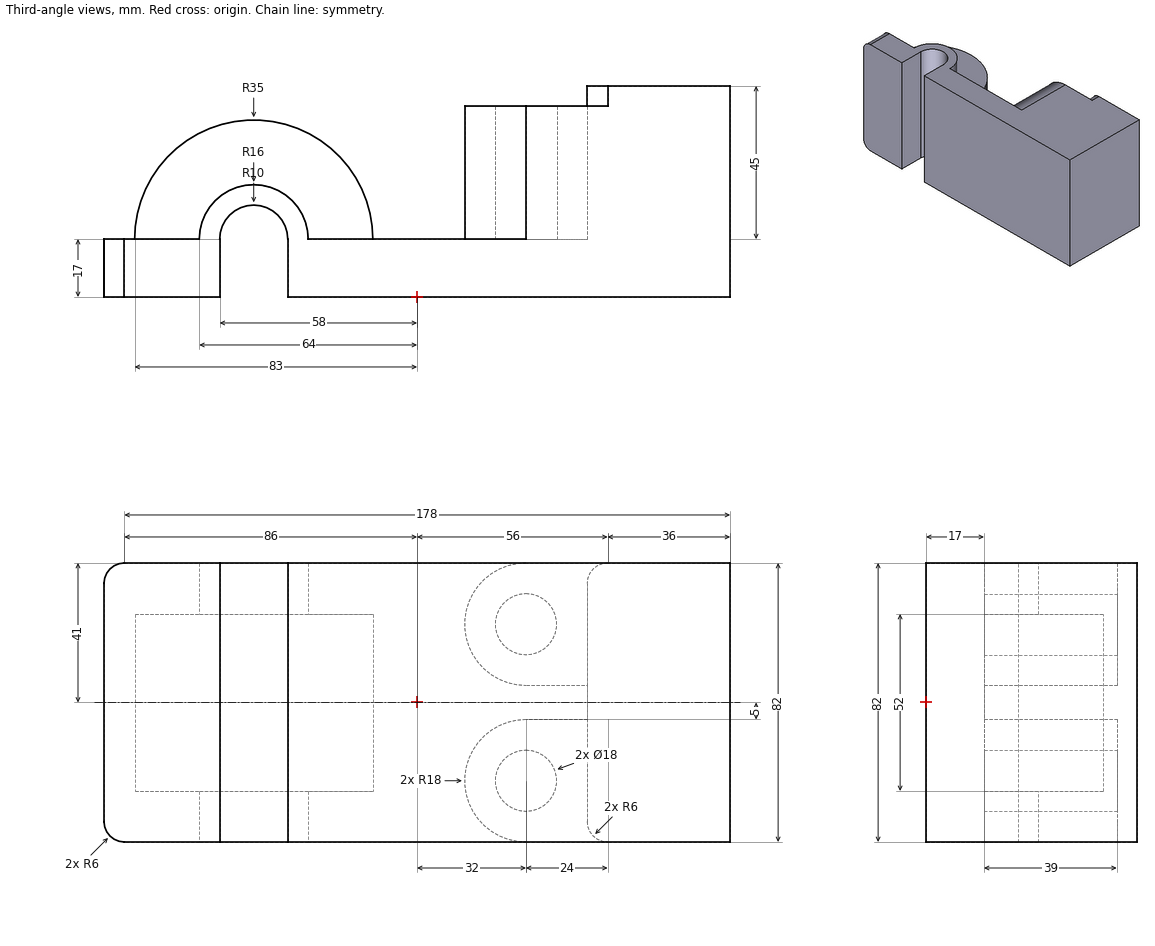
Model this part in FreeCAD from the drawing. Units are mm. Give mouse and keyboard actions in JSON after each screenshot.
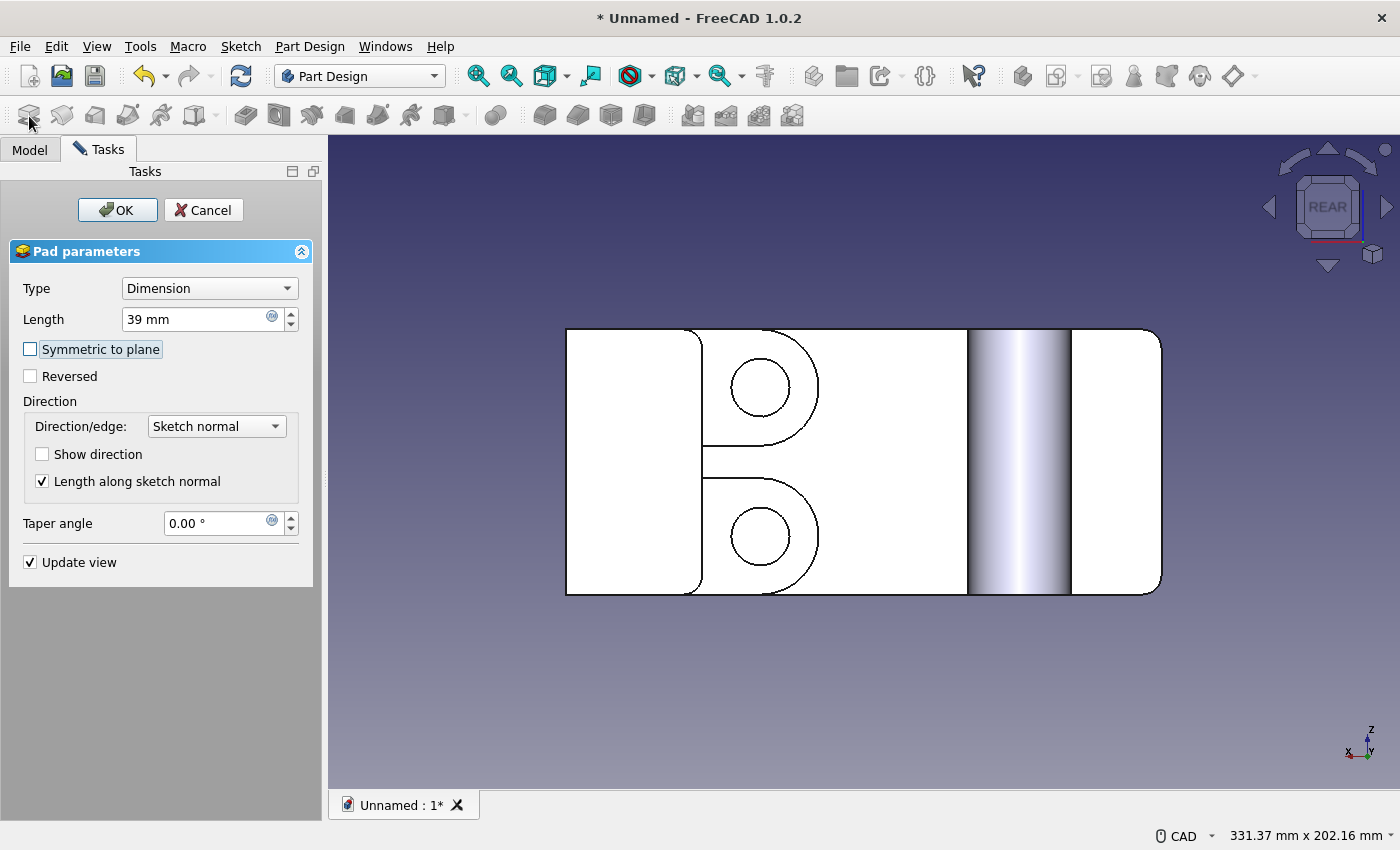
{"action": "left_click", "coordinate": [118, 210]}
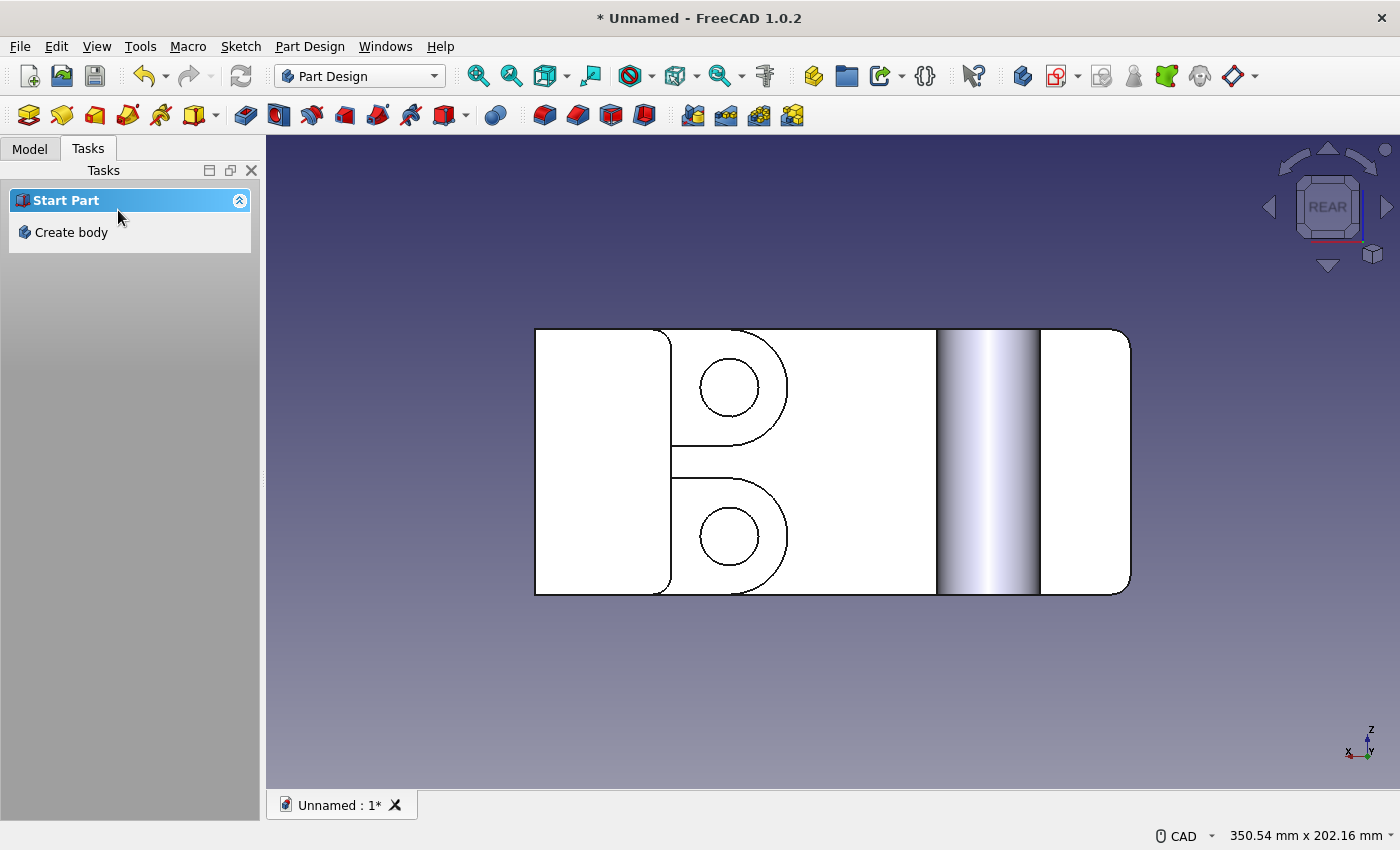
{"action": "left_click", "coordinate": [1056, 76]}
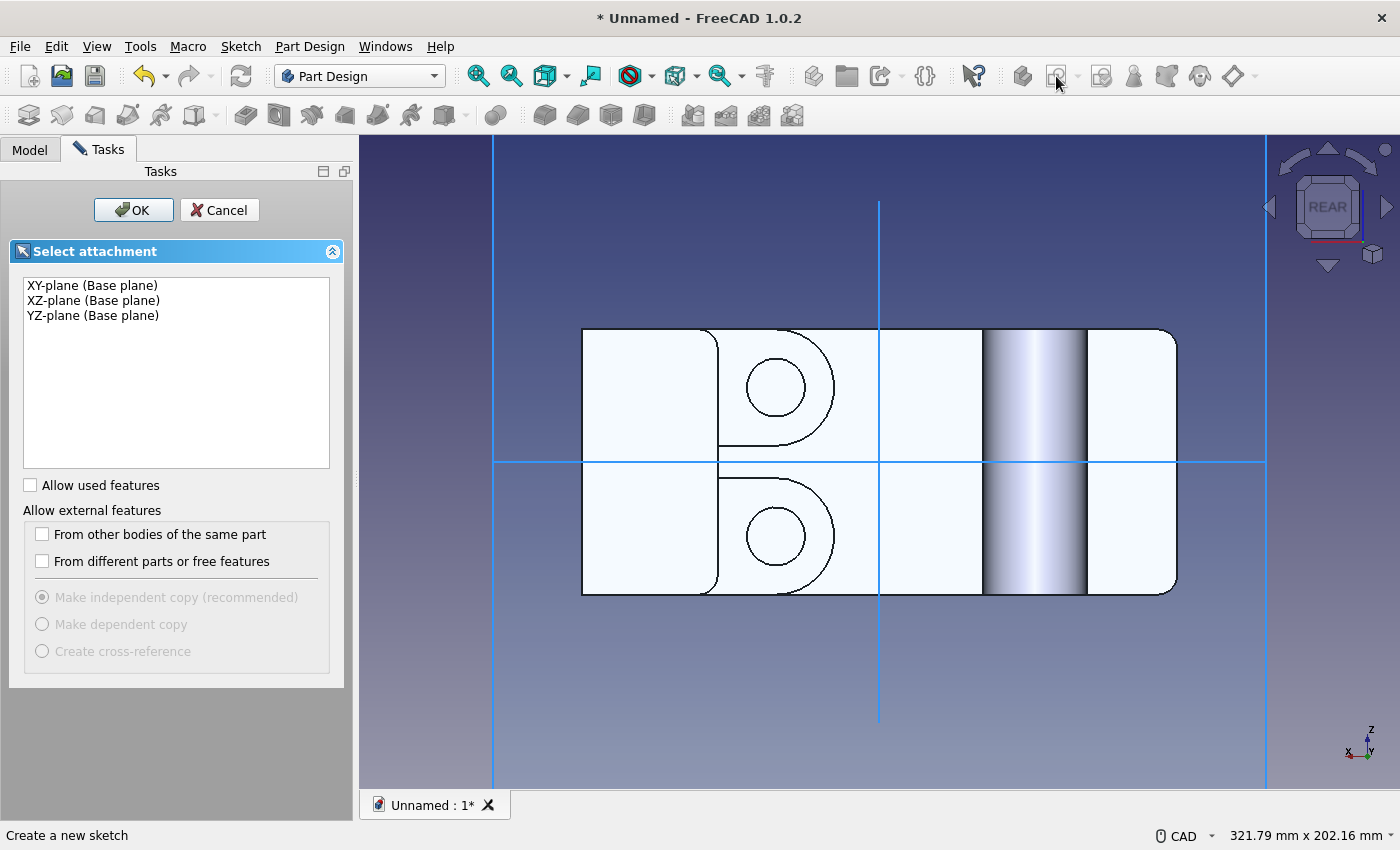
{"action": "left_click", "coordinate": [84, 286]}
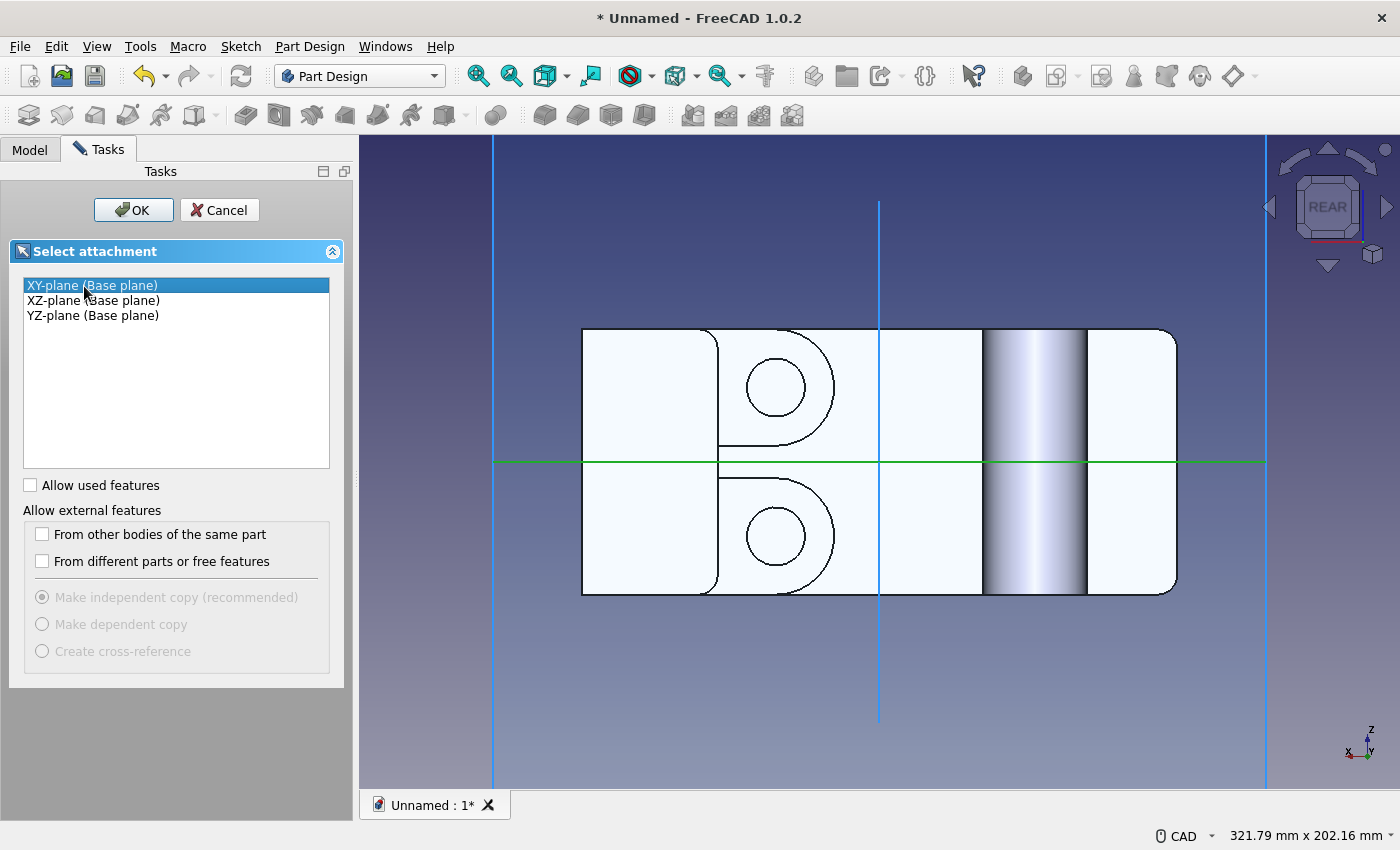
{"action": "left_click", "coordinate": [134, 210]}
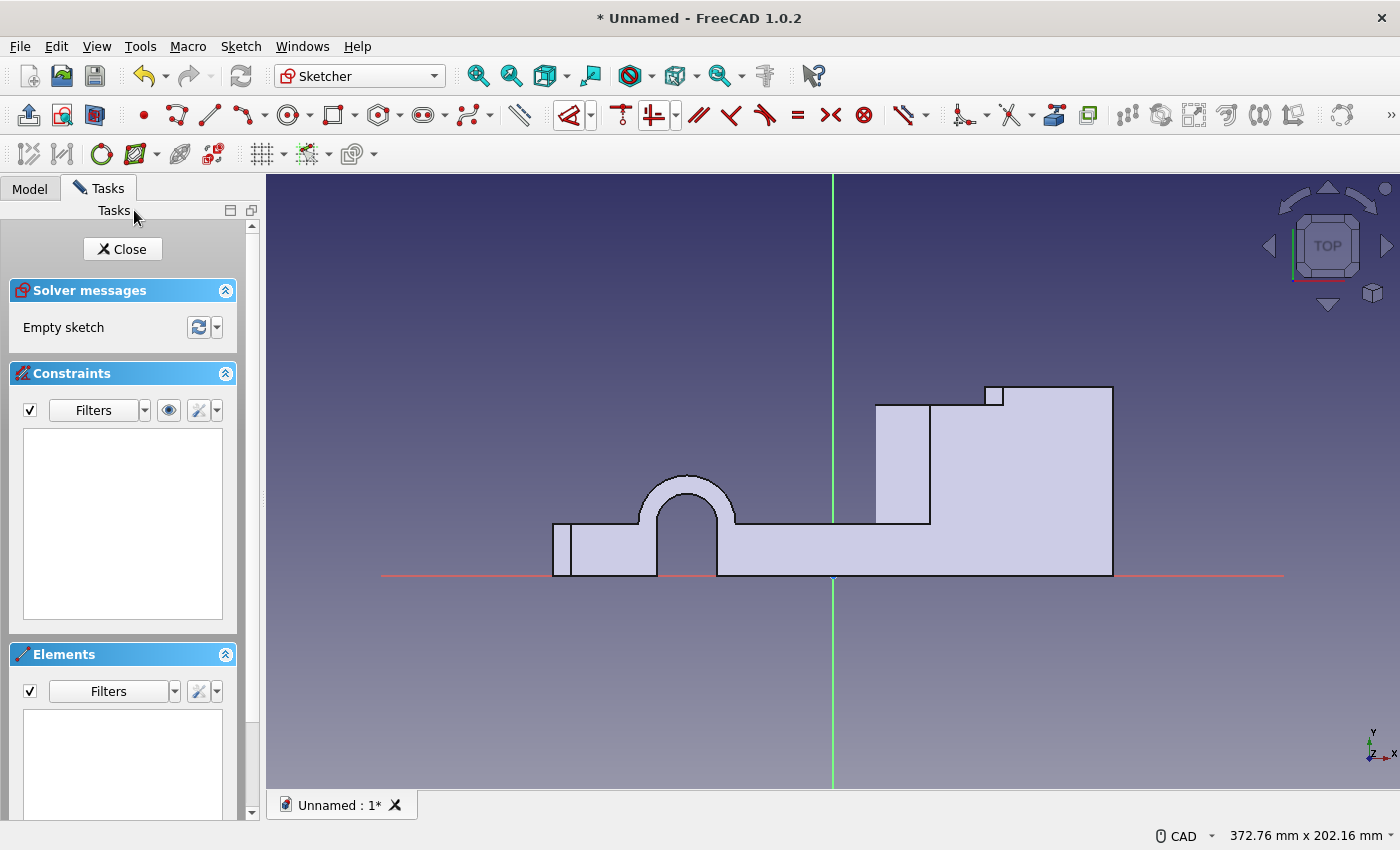
{"action": "left_click", "coordinate": [95, 116]}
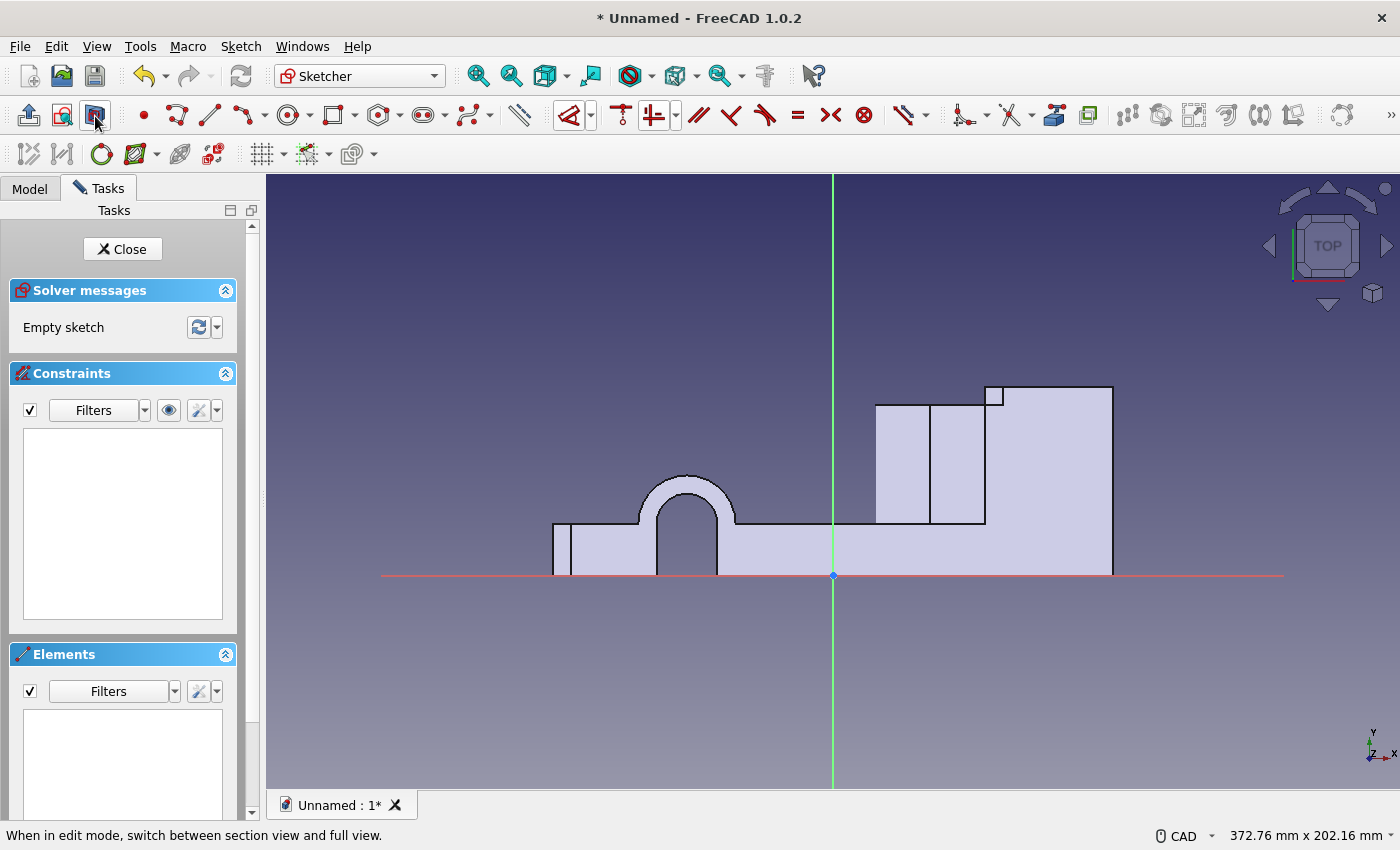
{"action": "scroll", "coordinate": [673, 506], "scroll_direction": "up", "scroll_amount": 5}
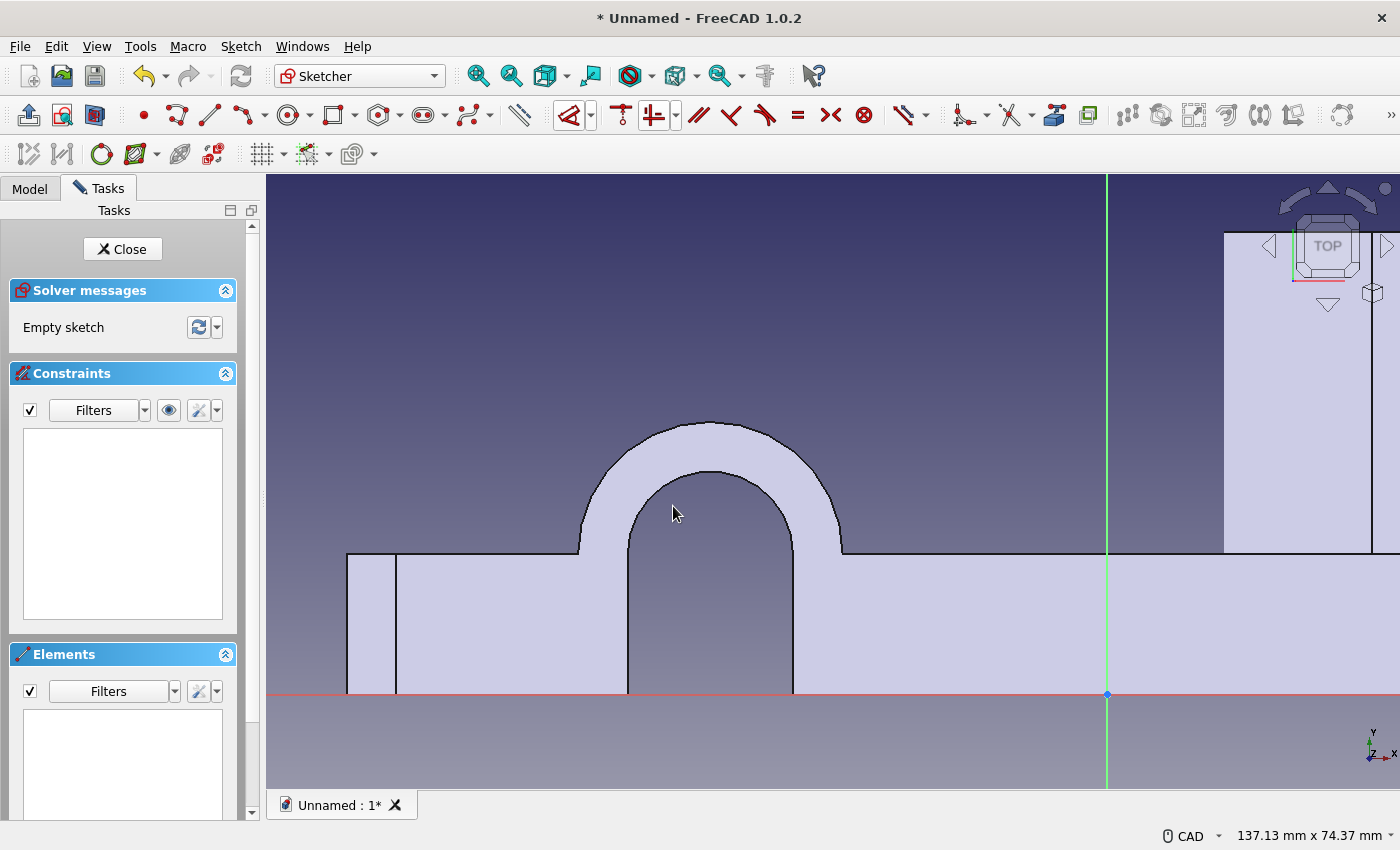
{"action": "left_click", "coordinate": [210, 116]}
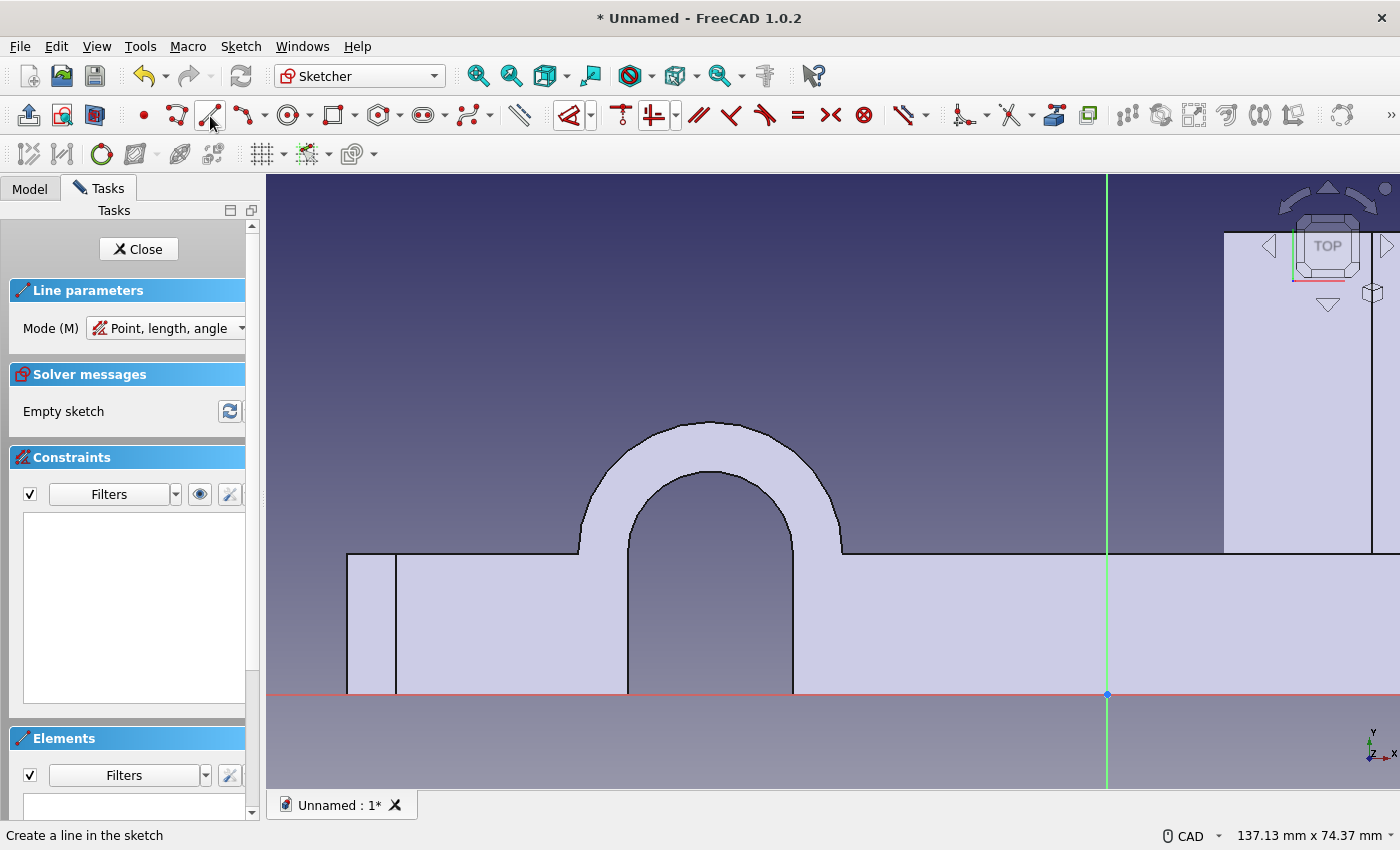
{"action": "left_click", "coordinate": [421, 554]}
{"action": "left_click", "coordinate": [578, 554]}